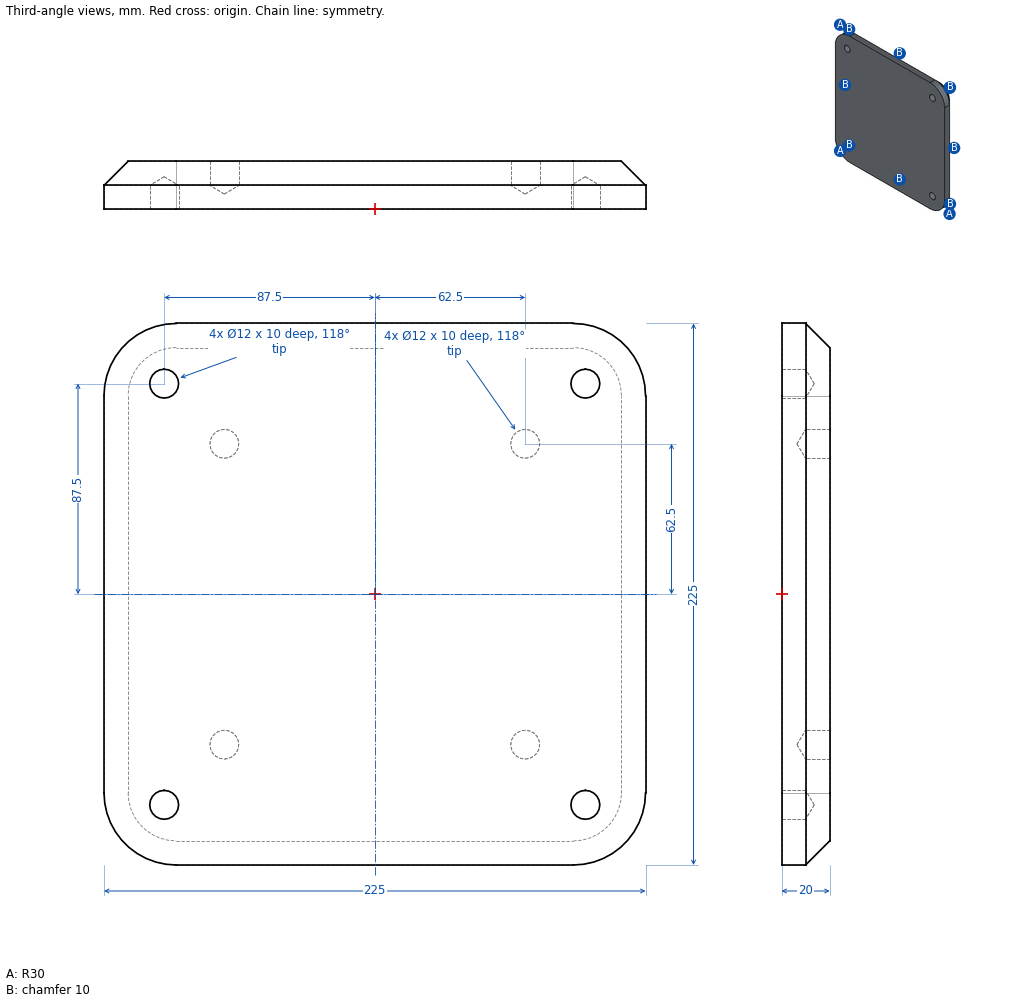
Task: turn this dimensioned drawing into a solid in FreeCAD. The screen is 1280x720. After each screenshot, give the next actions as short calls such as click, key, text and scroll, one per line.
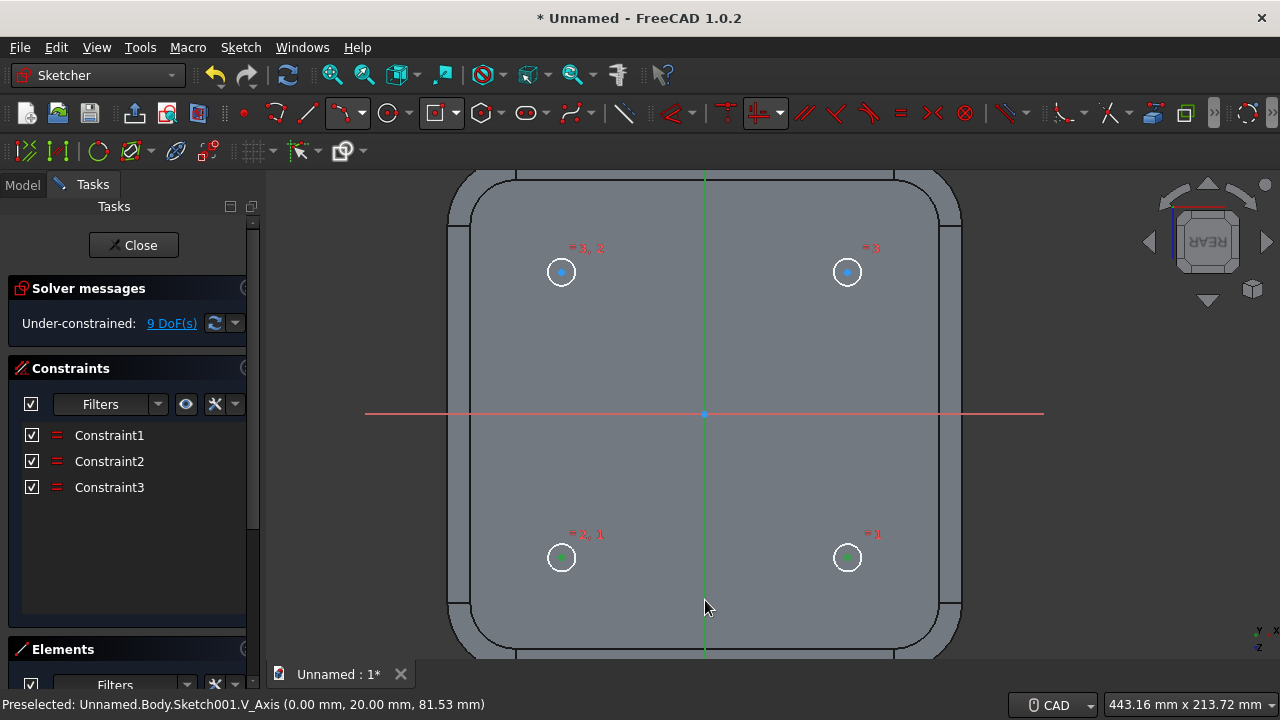
key(s)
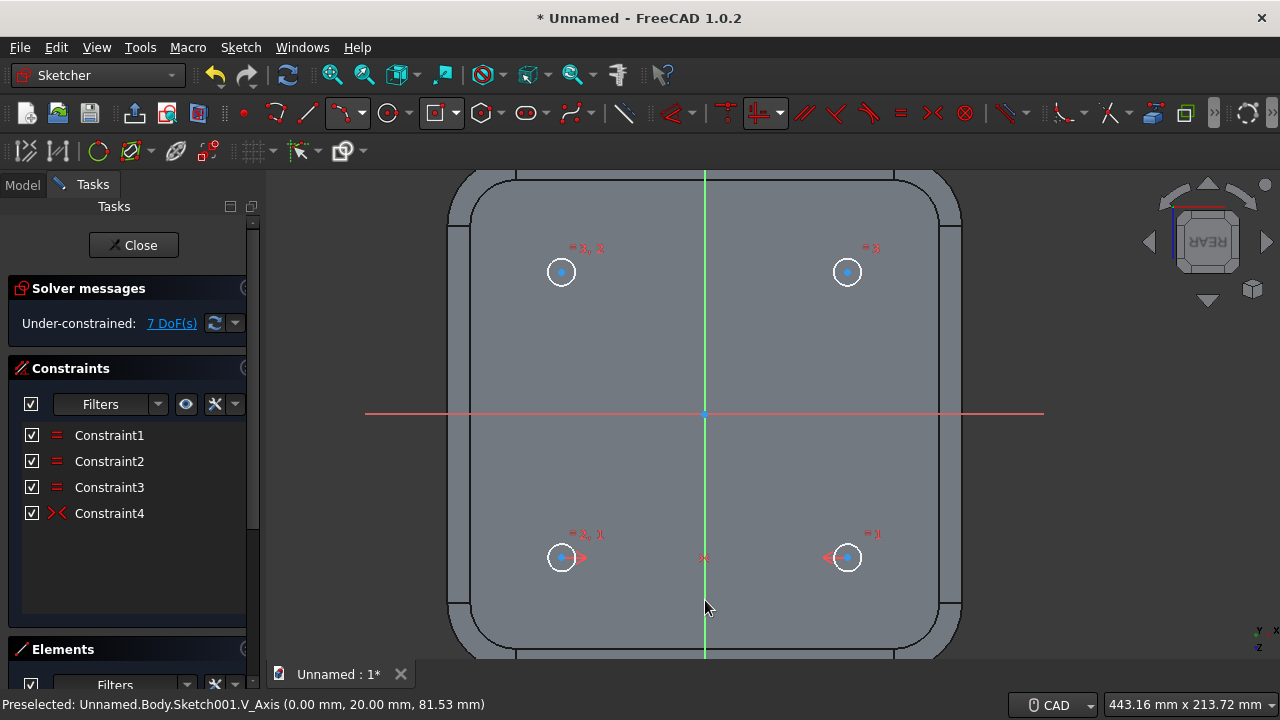
click(562, 558)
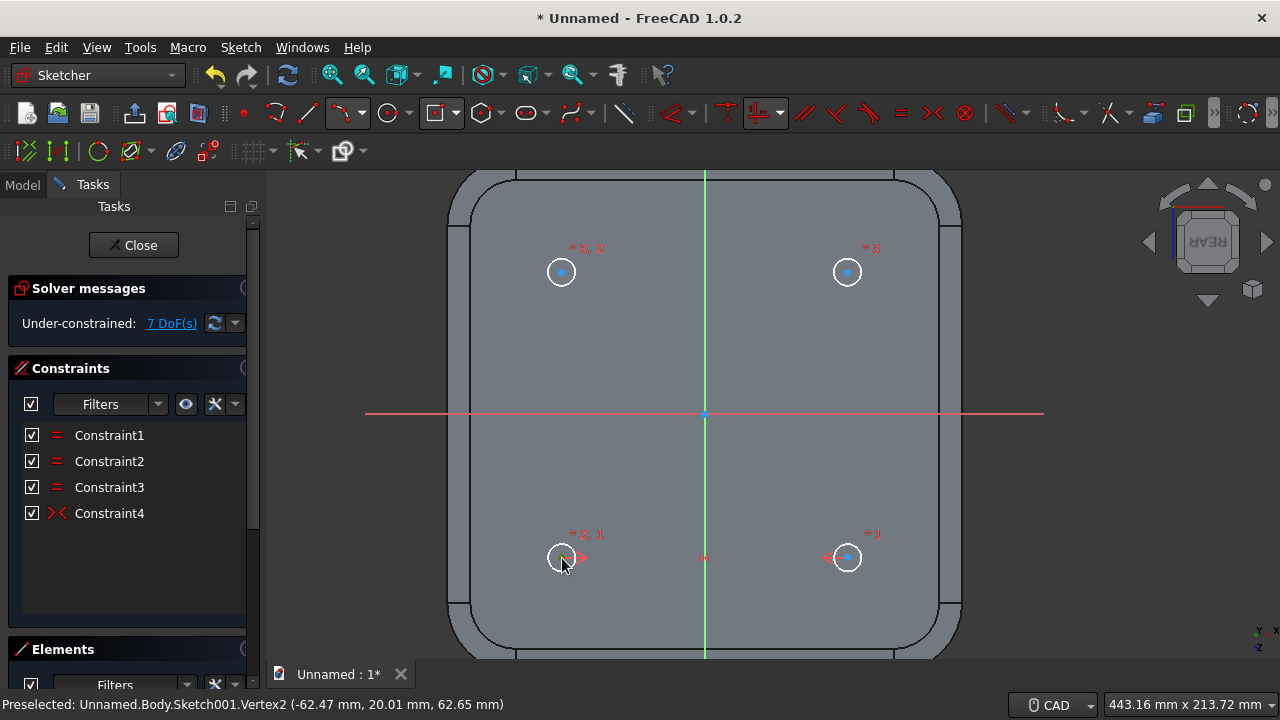
click(562, 272)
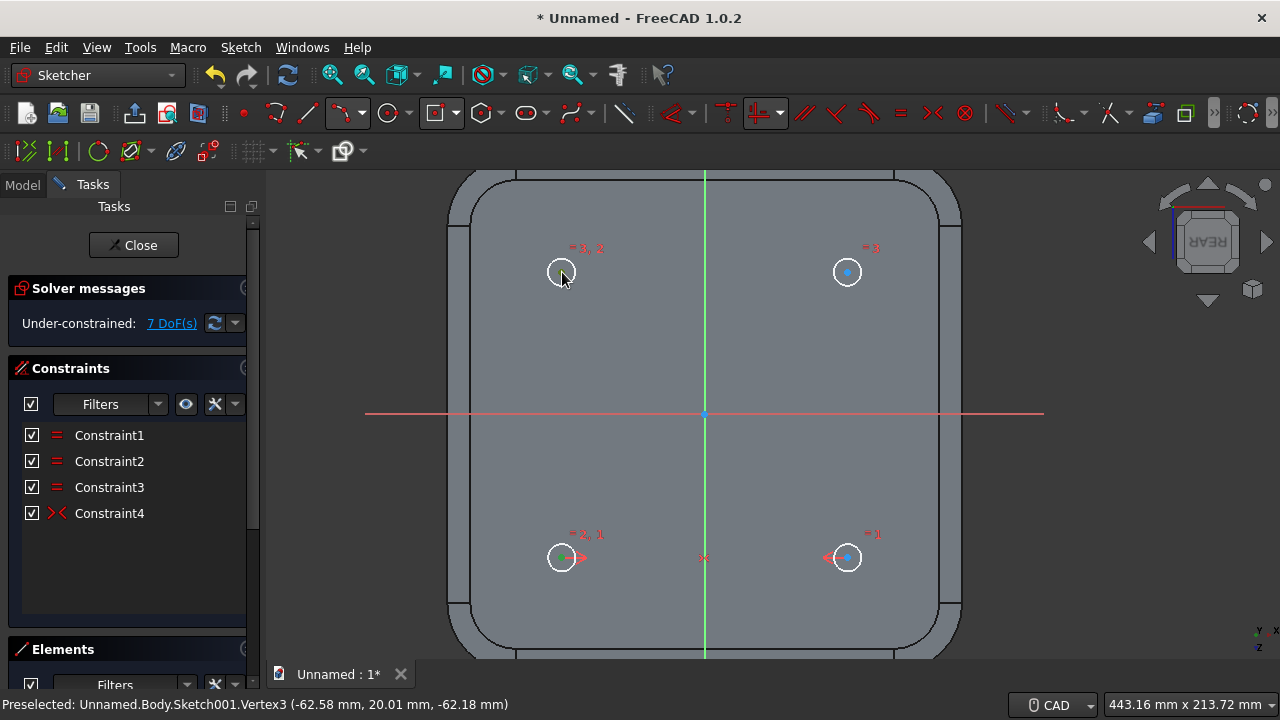
click(411, 414)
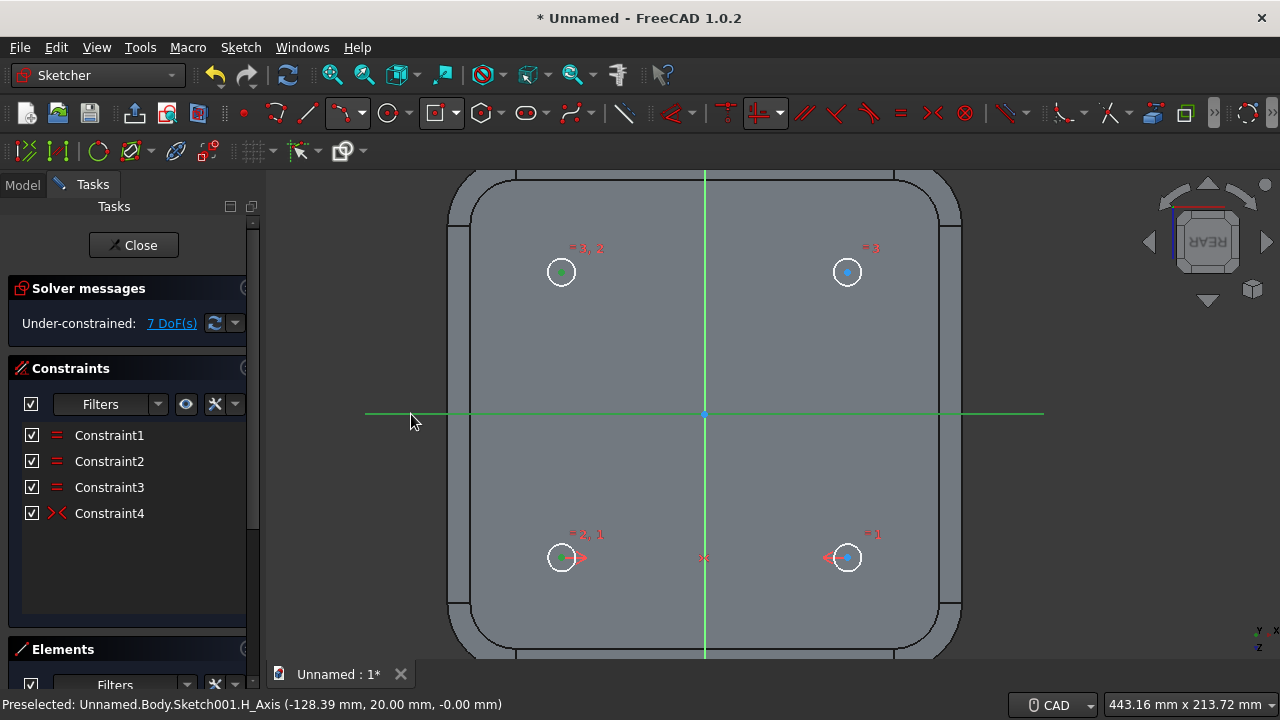
click(934, 114)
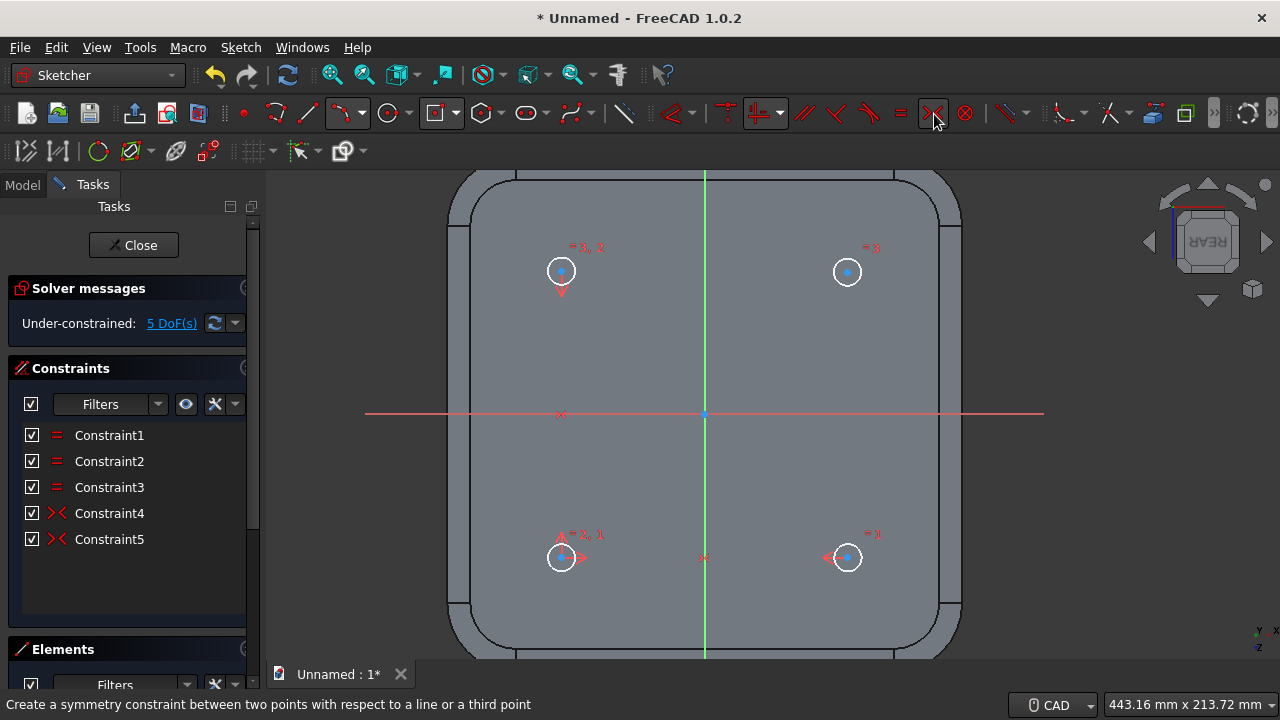
click(848, 558)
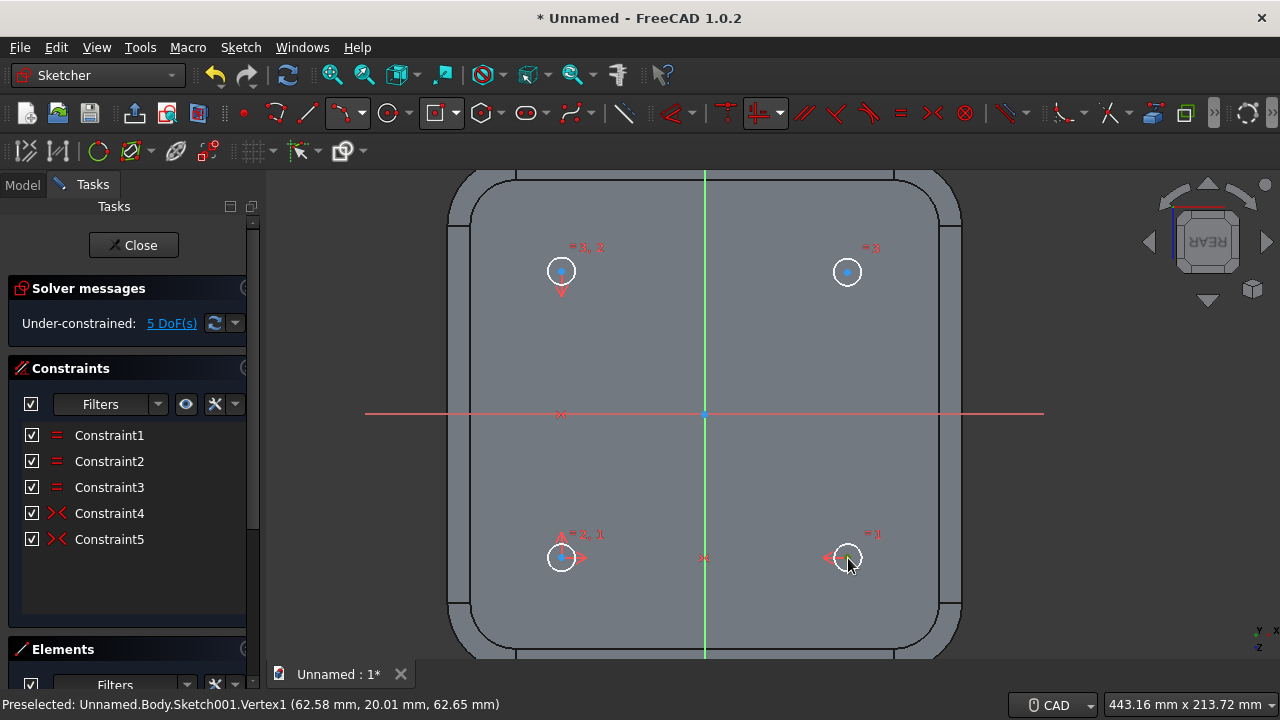
click(848, 272)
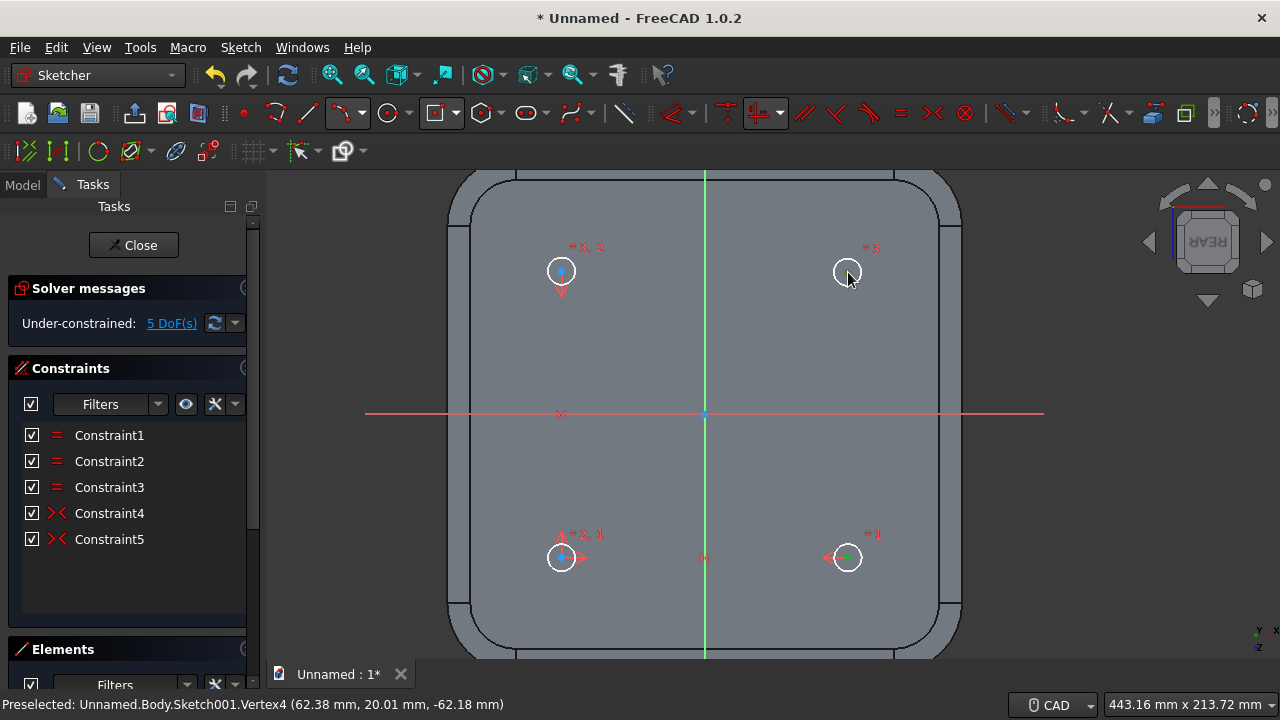
click(411, 414)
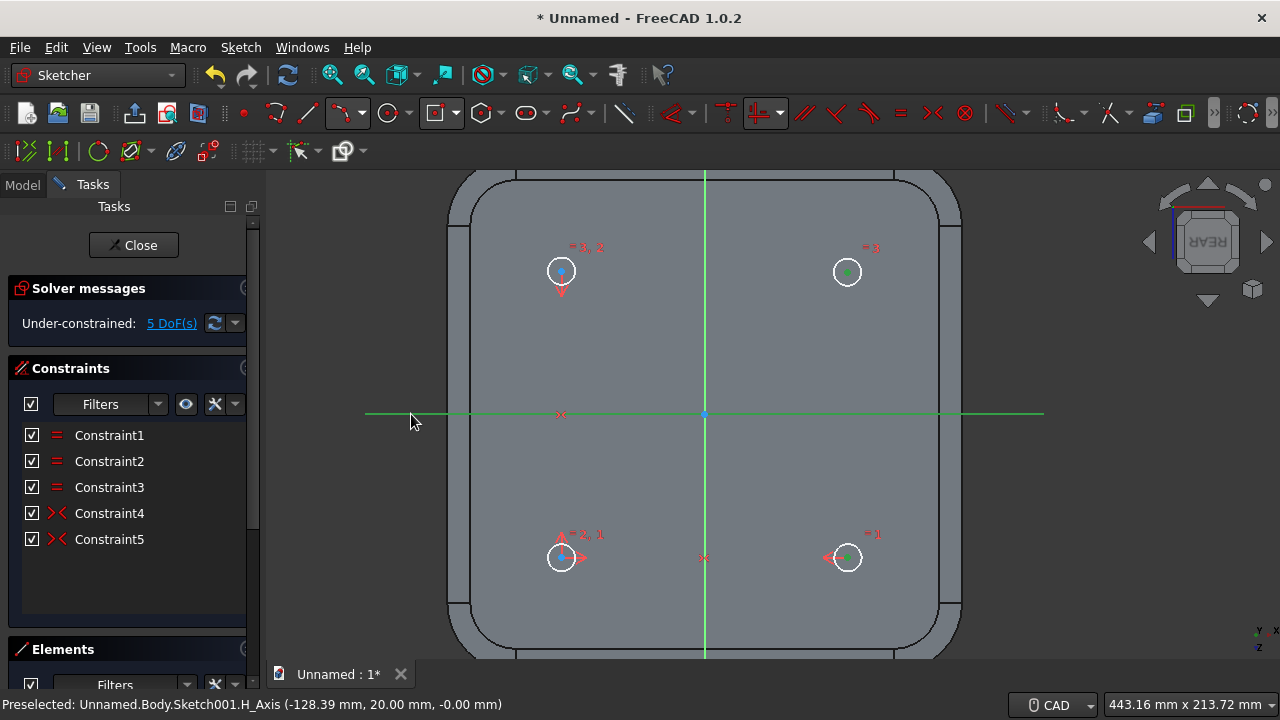
click(934, 114)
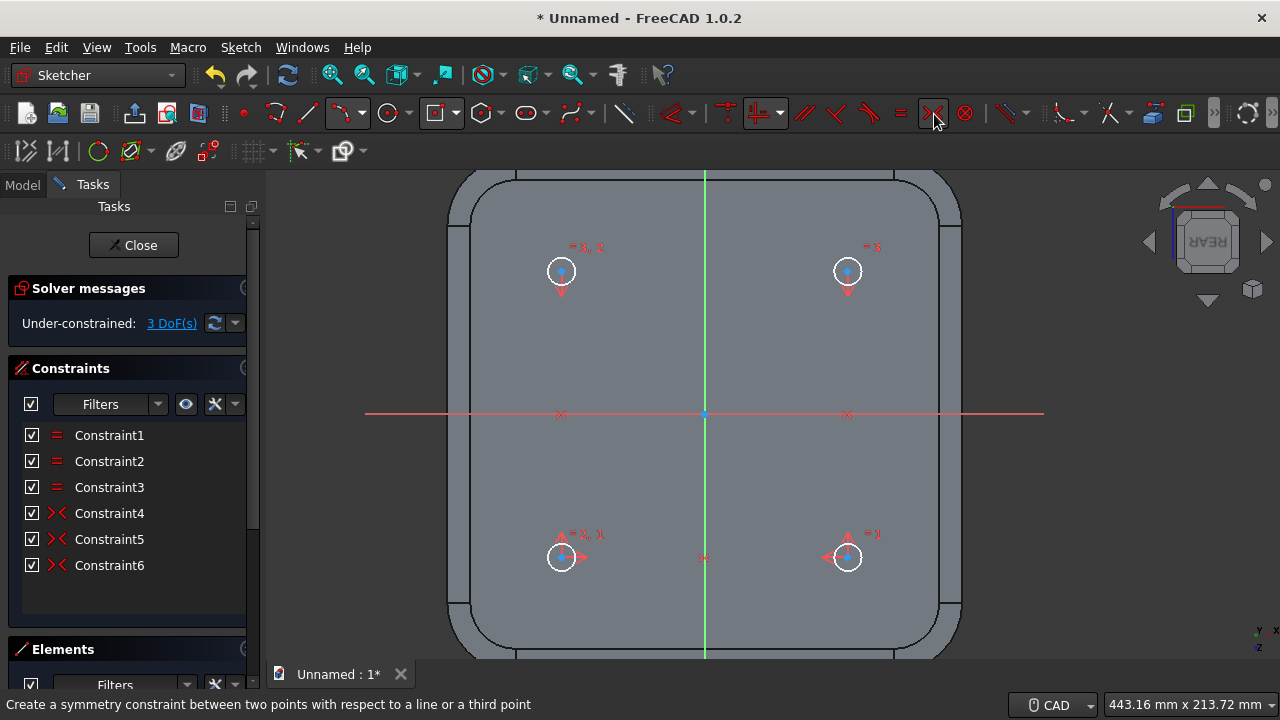
key(d)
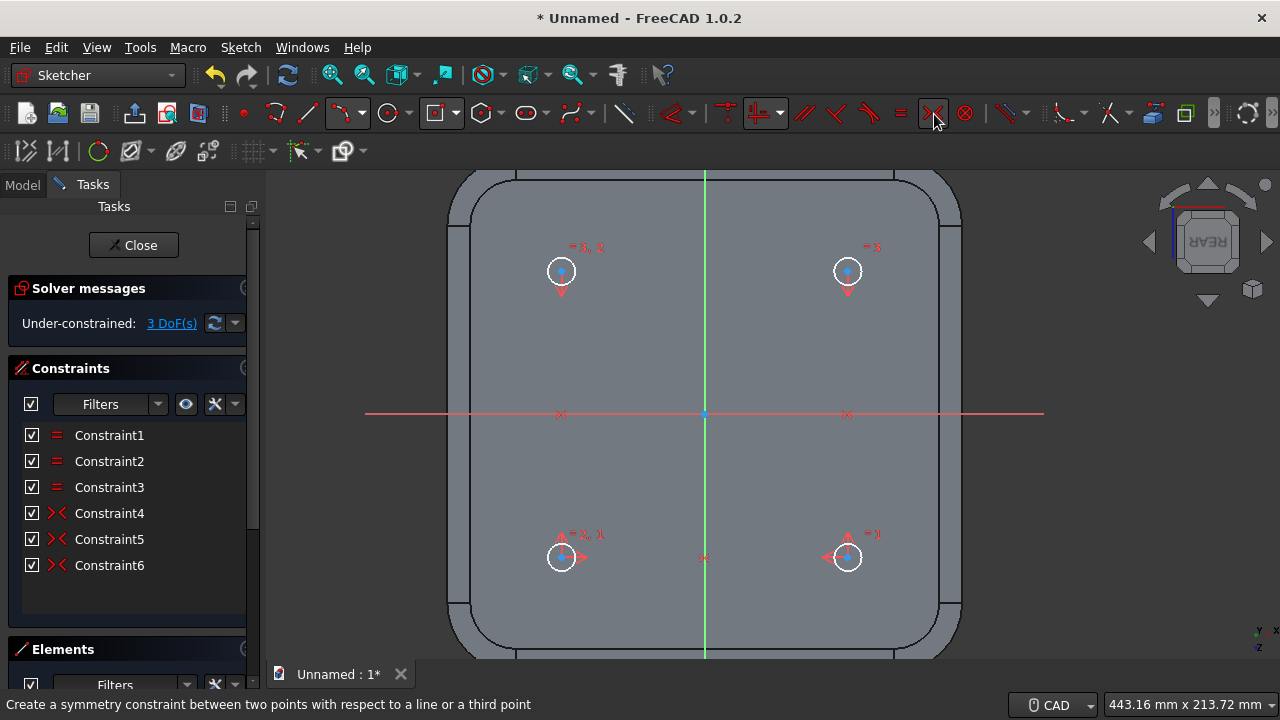
scroll(858, 548, up, 2)